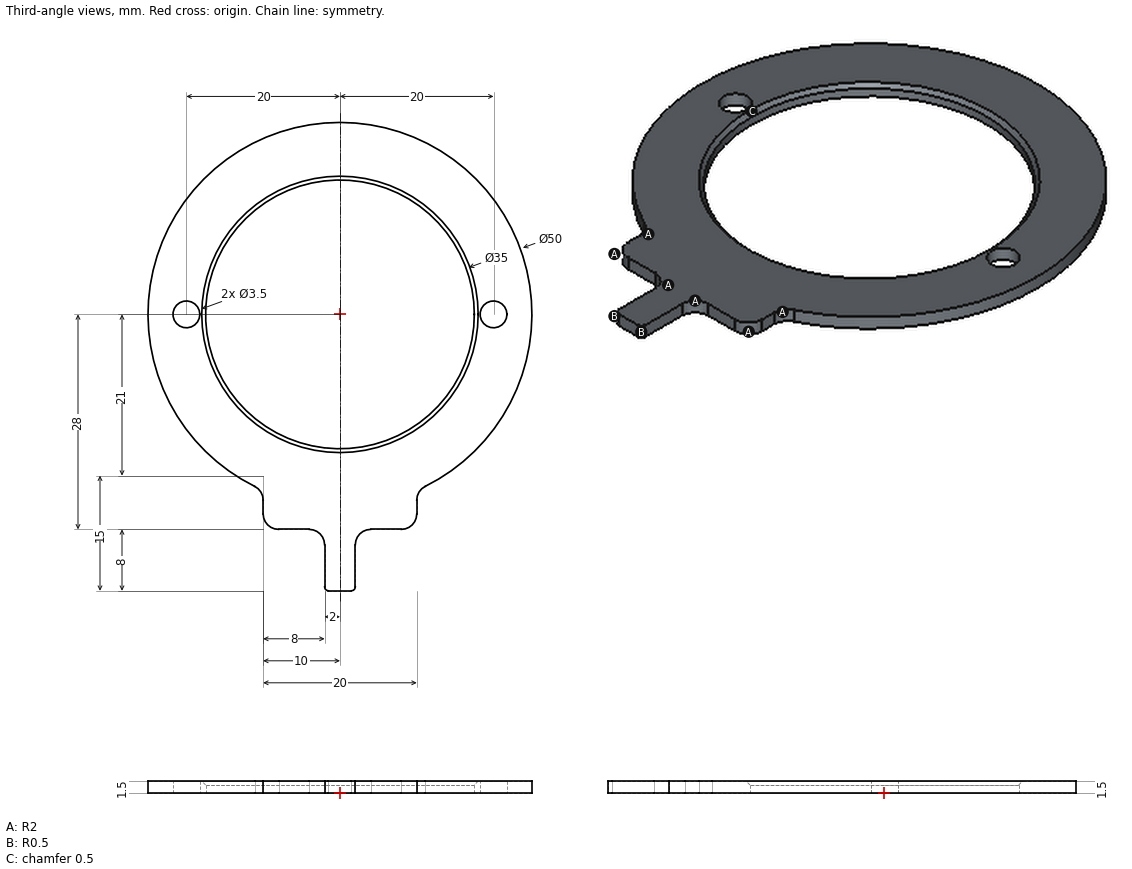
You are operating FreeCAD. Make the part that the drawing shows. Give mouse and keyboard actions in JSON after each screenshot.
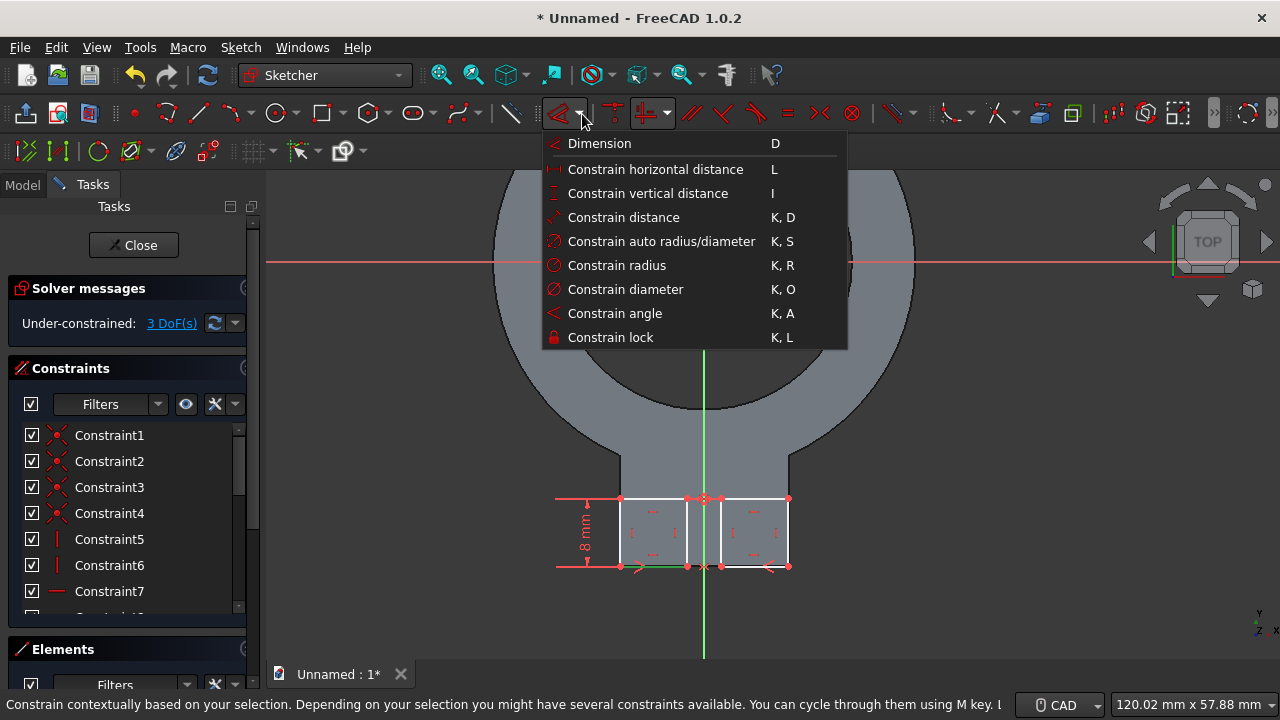
{"action": "left_click", "coordinate": [695, 169]}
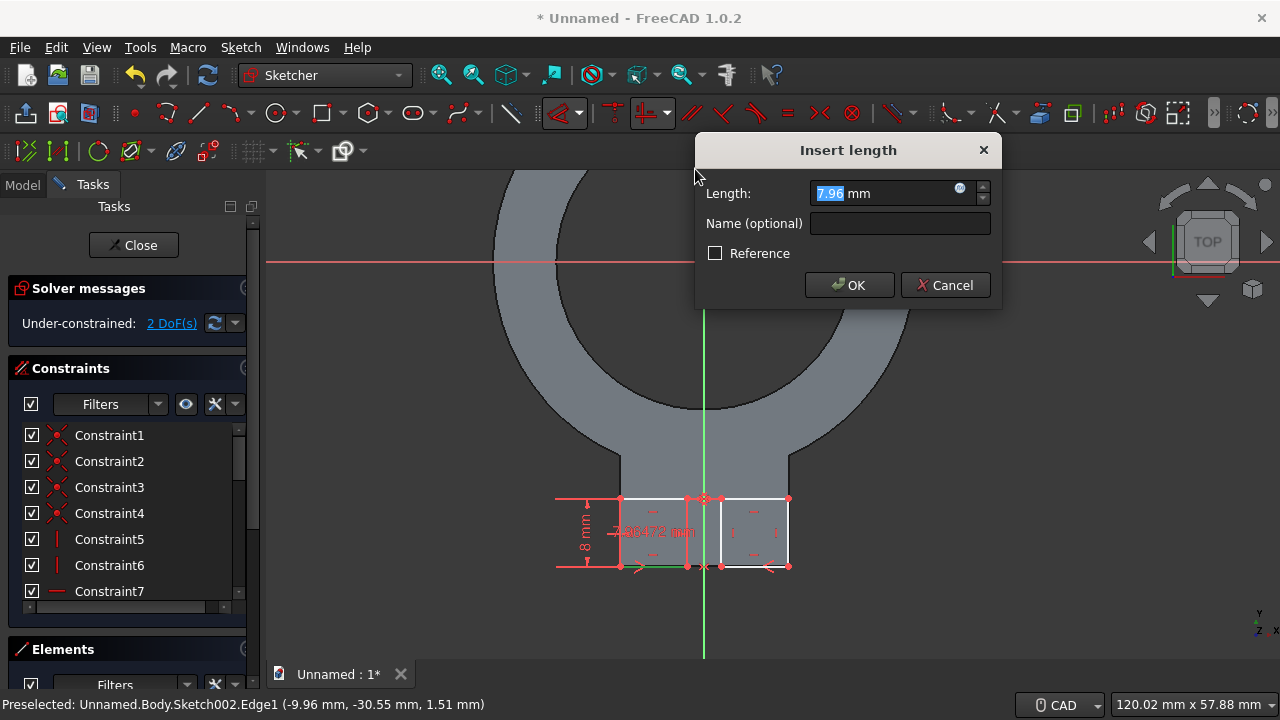
{"action": "type", "text": "8"}
{"action": "key", "text": "Return"}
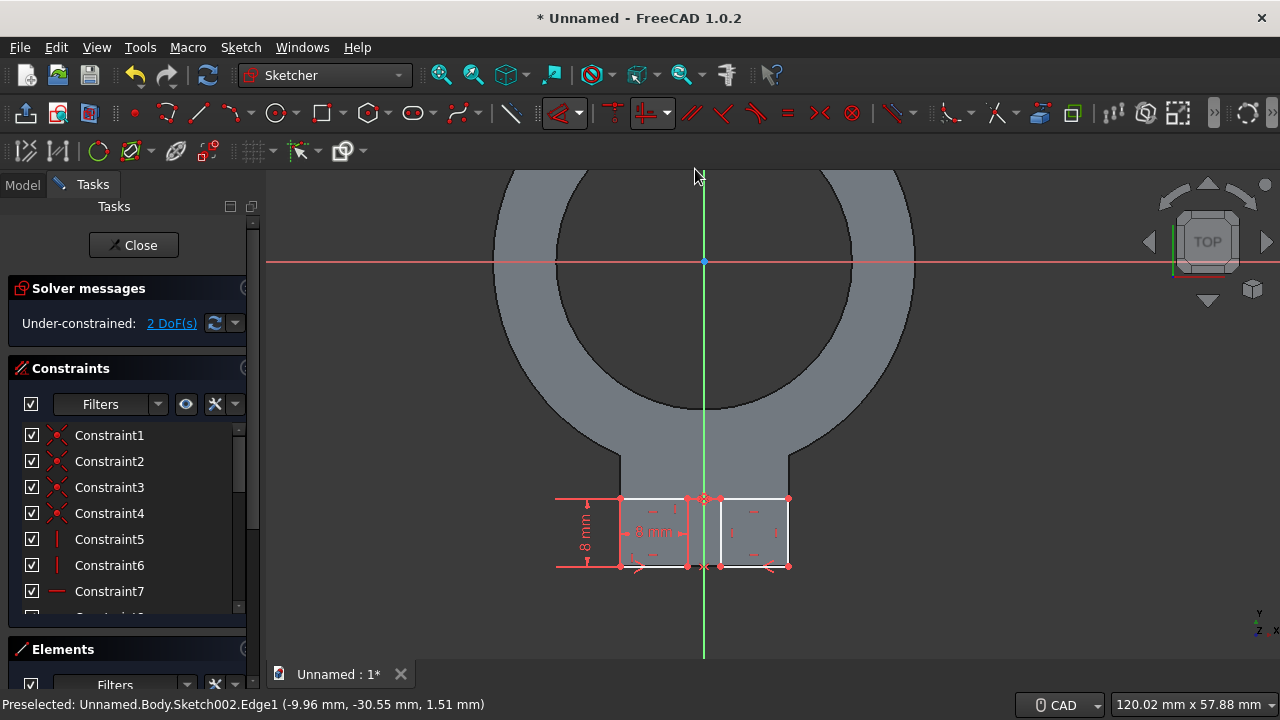
{"action": "scroll", "coordinate": [688, 567], "scroll_direction": "up", "scroll_amount": 5}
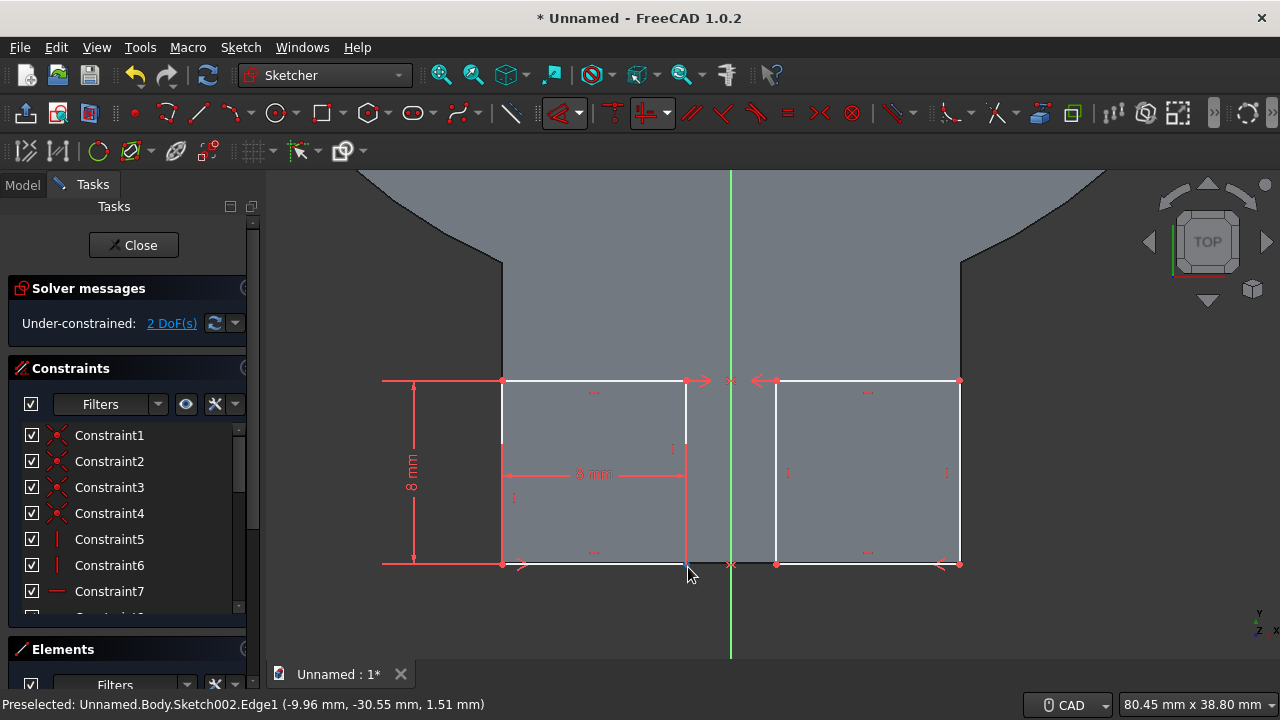
{"action": "left_click", "coordinate": [686, 564]}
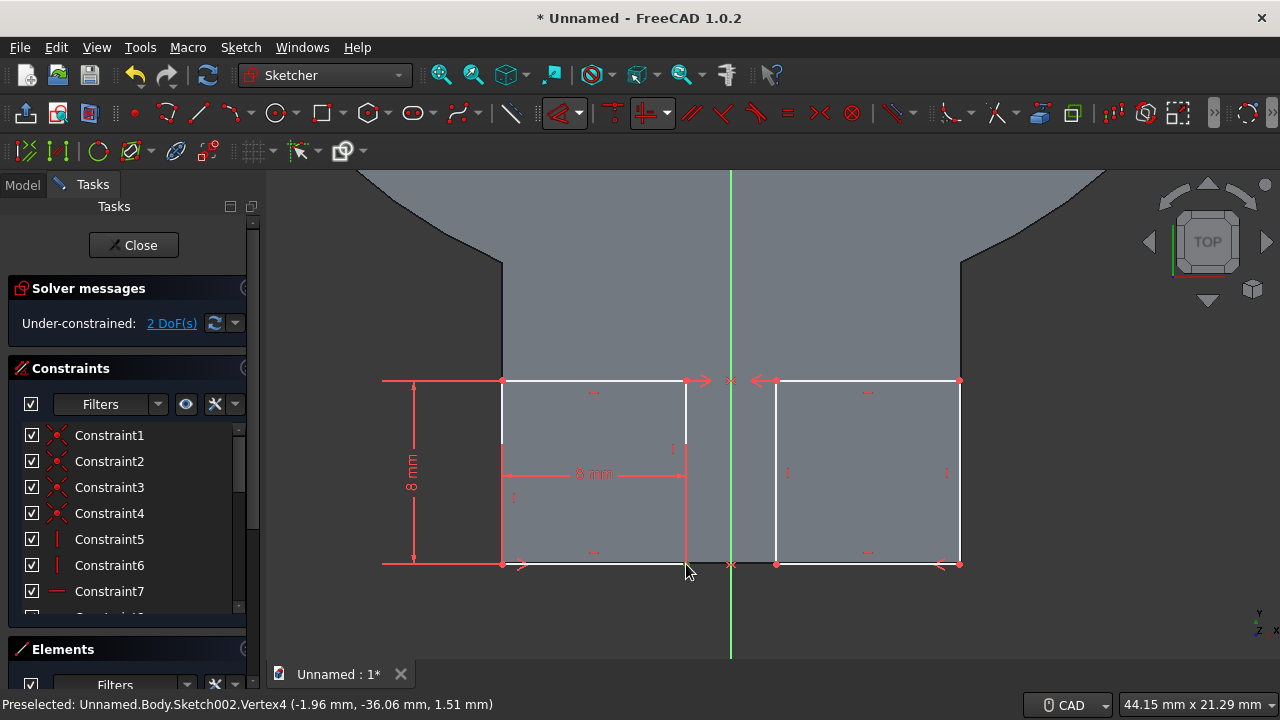
{"action": "left_click", "coordinate": [582, 114]}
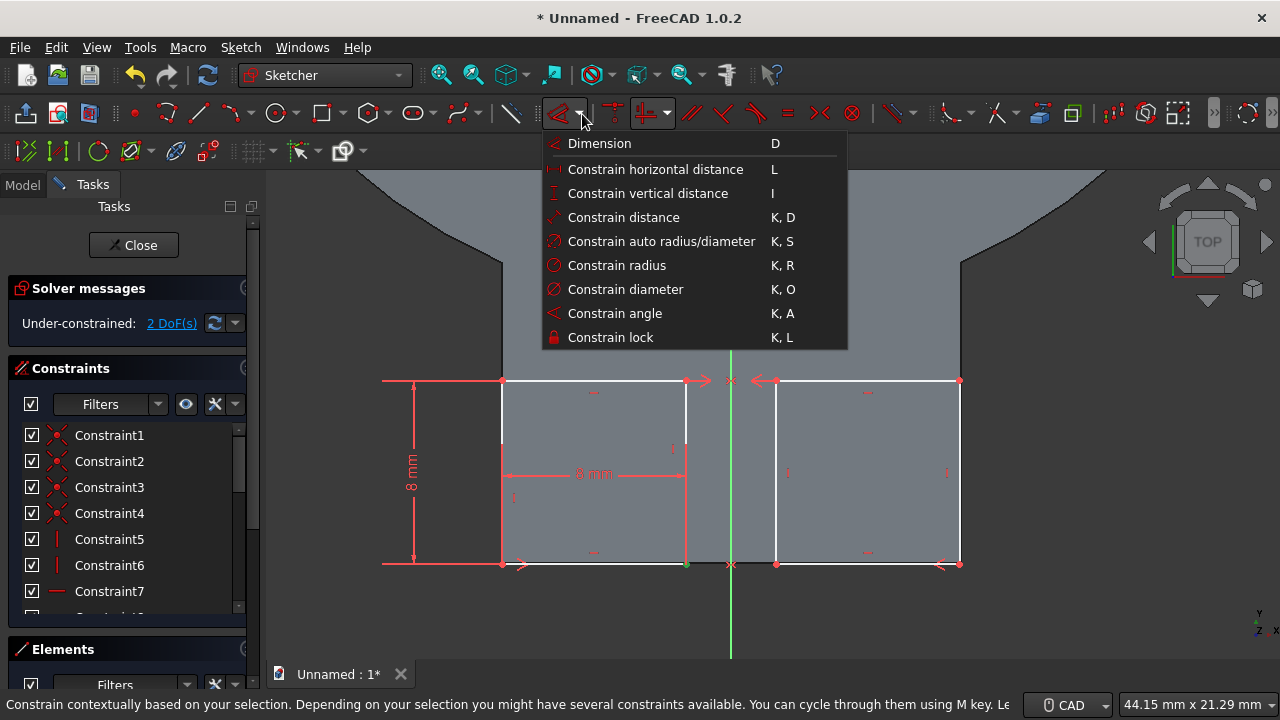
{"action": "left_click", "coordinate": [695, 169]}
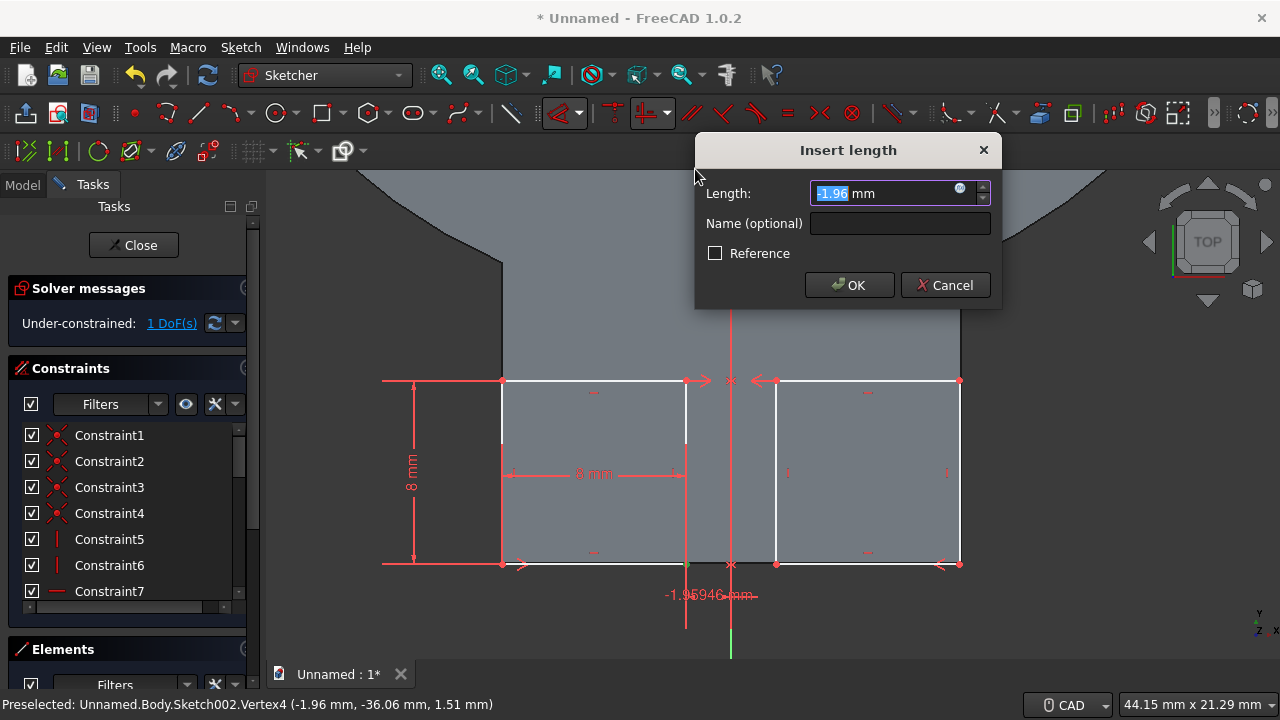
{"action": "type", "text": "-2"}
{"action": "key", "text": "Return"}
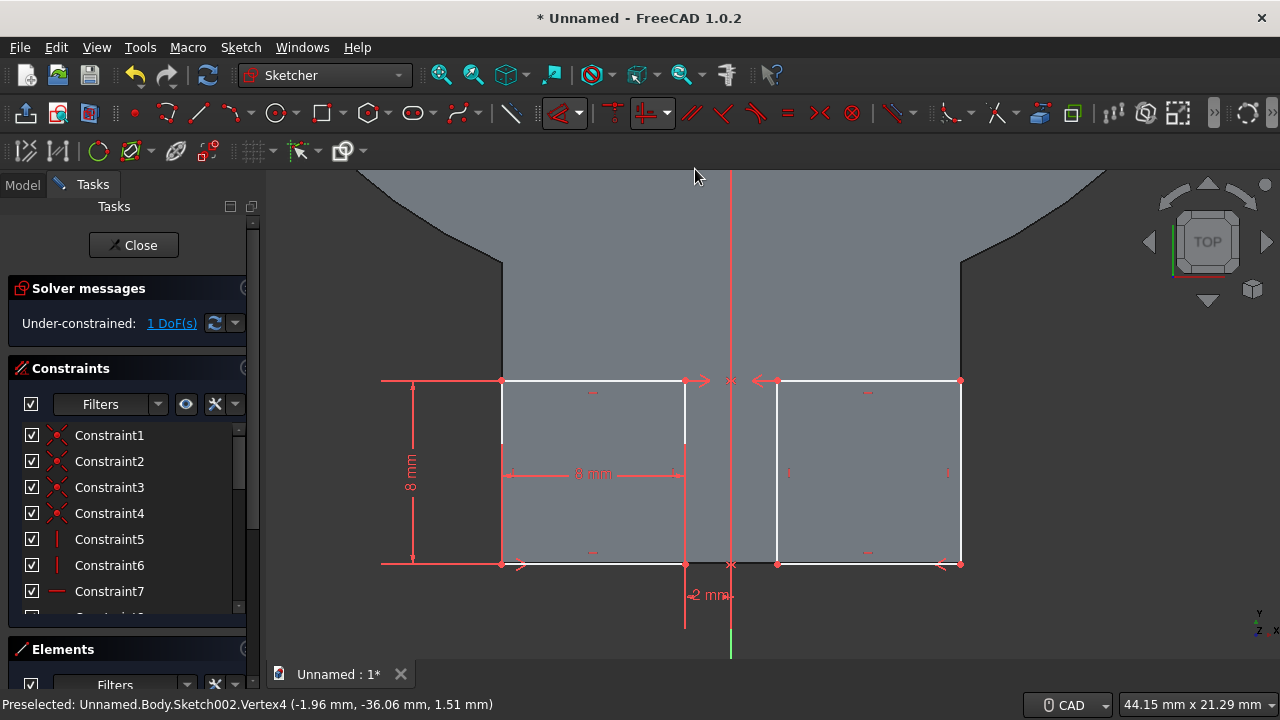
{"action": "left_click", "coordinate": [502, 381]}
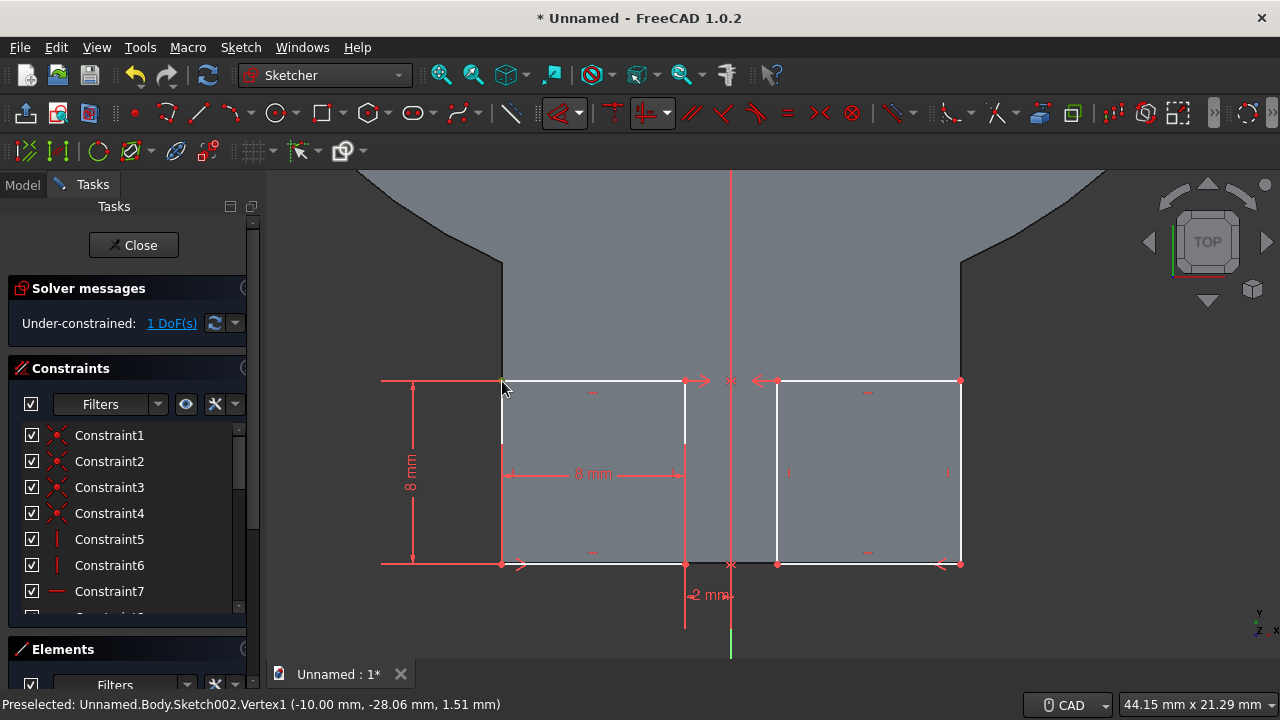
{"action": "left_click", "coordinate": [582, 114]}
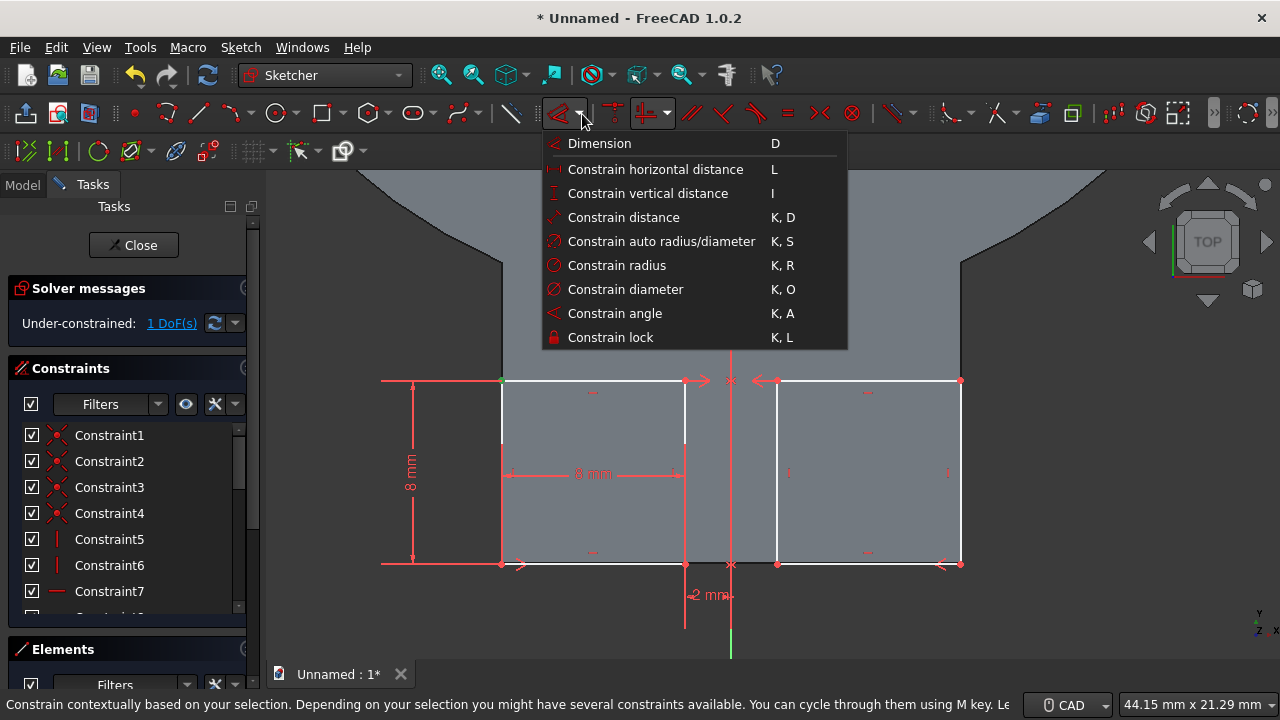
{"action": "left_click", "coordinate": [695, 193]}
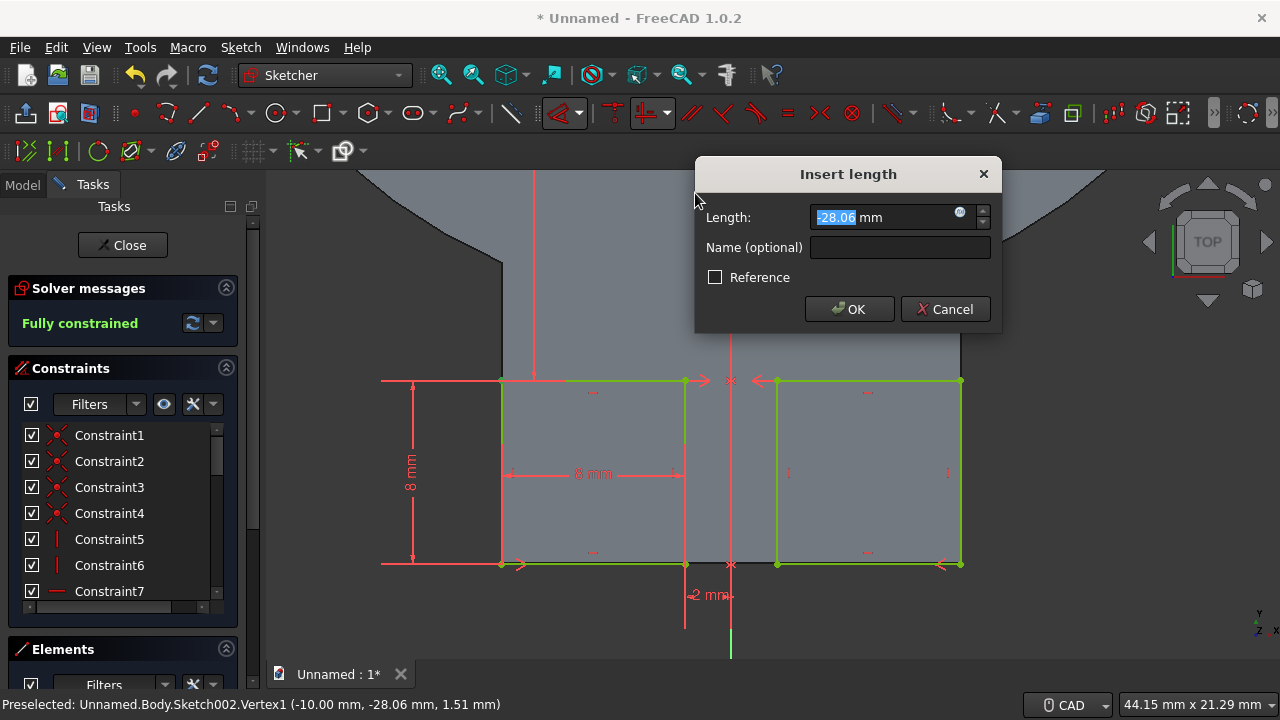
{"action": "type", "text": "-28"}
{"action": "key", "text": "Return"}